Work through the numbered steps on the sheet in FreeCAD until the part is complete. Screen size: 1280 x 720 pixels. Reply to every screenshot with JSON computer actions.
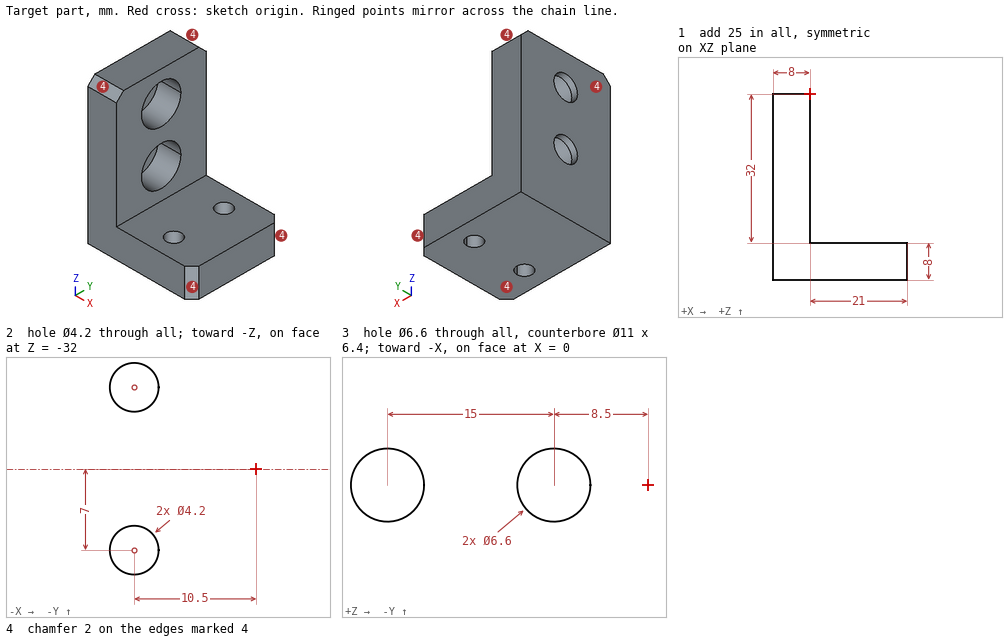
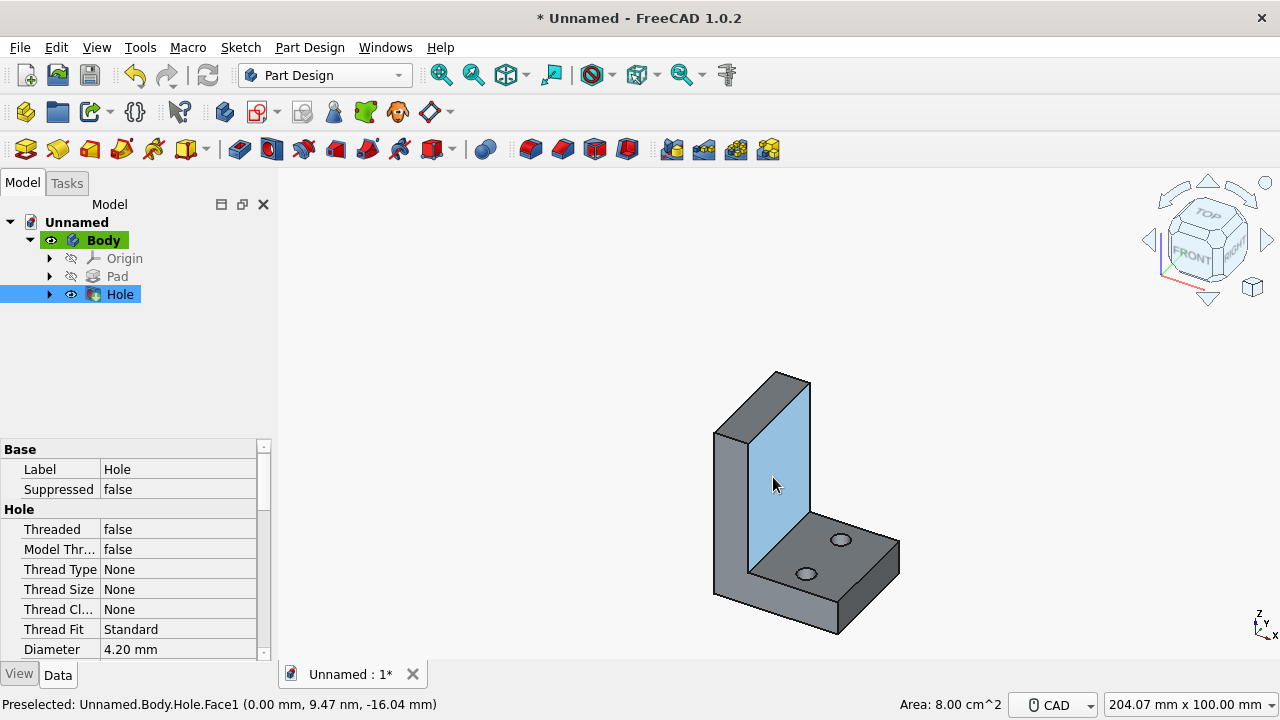
{"action": "left_click", "coordinate": [258, 112]}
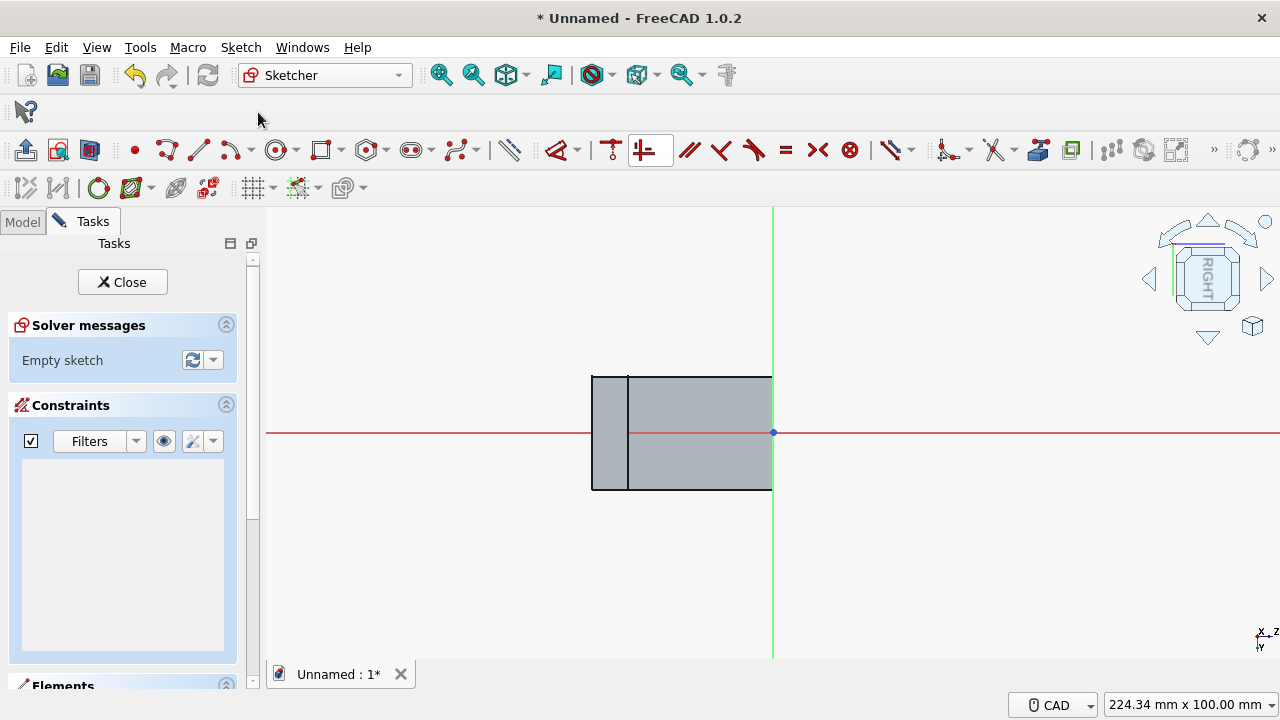
{"action": "left_click", "coordinate": [90, 150]}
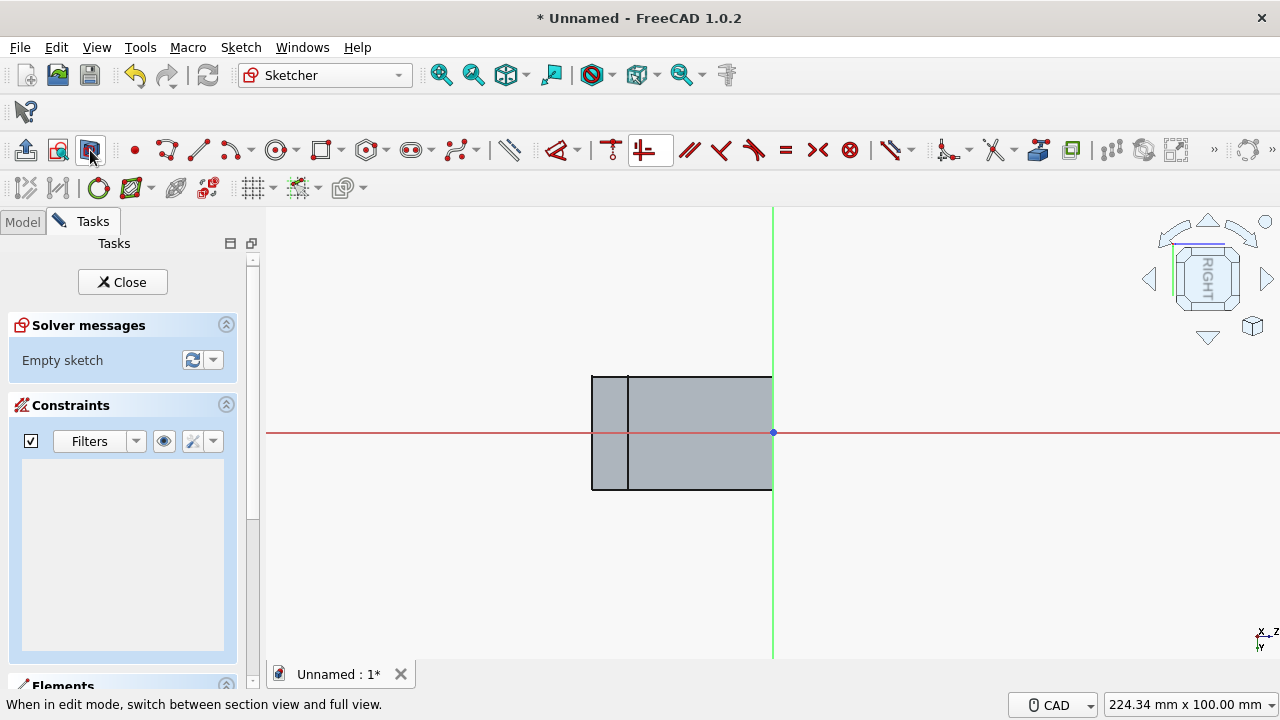
{"action": "scroll", "coordinate": [714, 433], "scroll_direction": "up", "scroll_amount": 8}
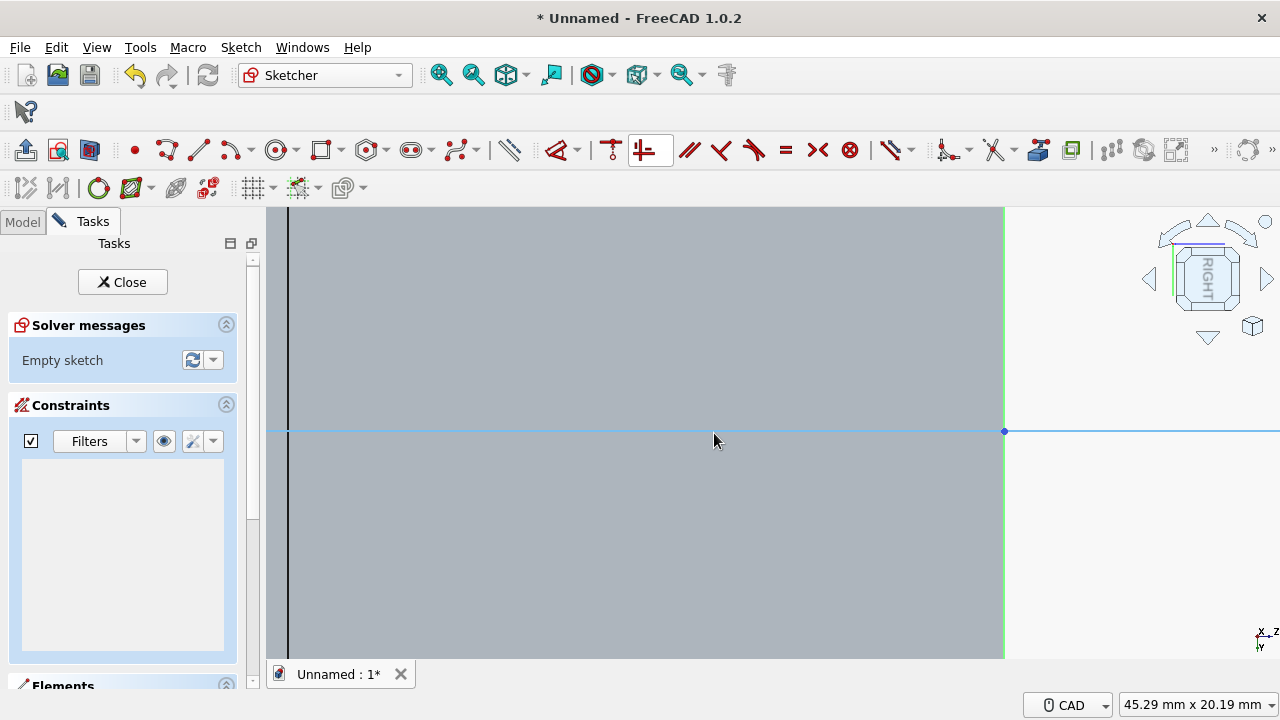
{"action": "key", "text": "g c"}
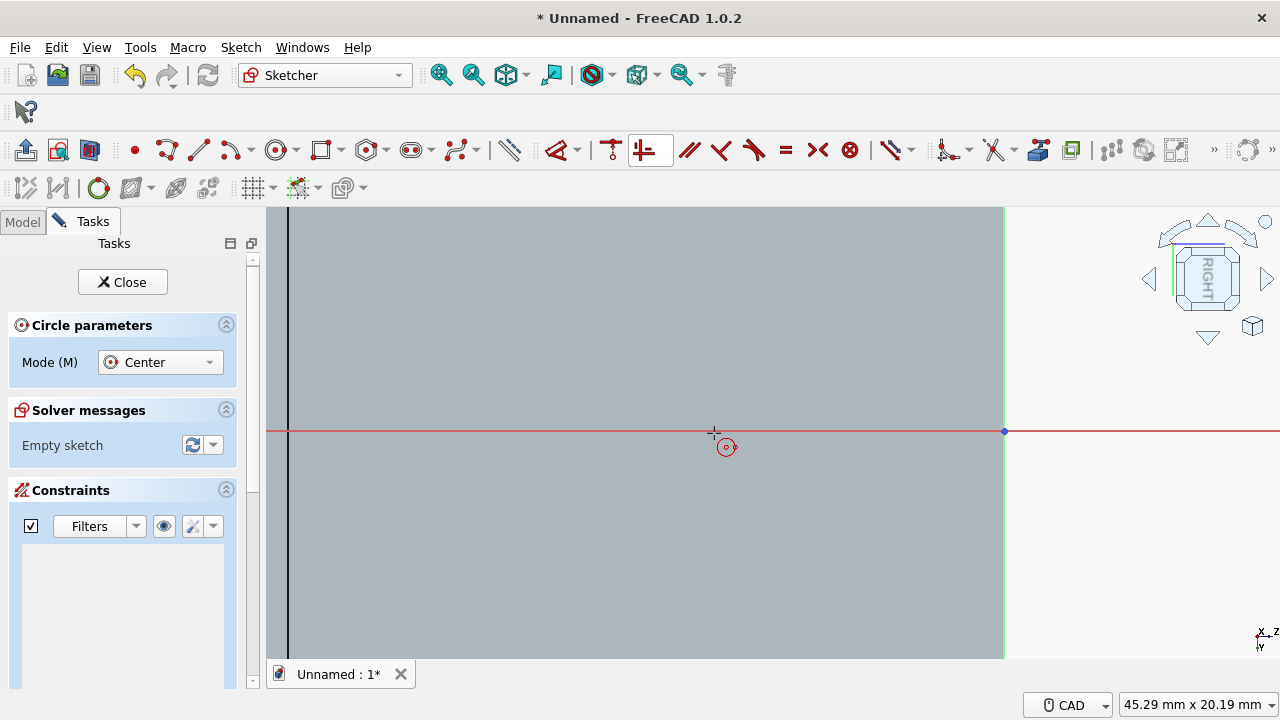
{"action": "left_click", "coordinate": [814, 431]}
{"action": "left_click", "coordinate": [866, 379]}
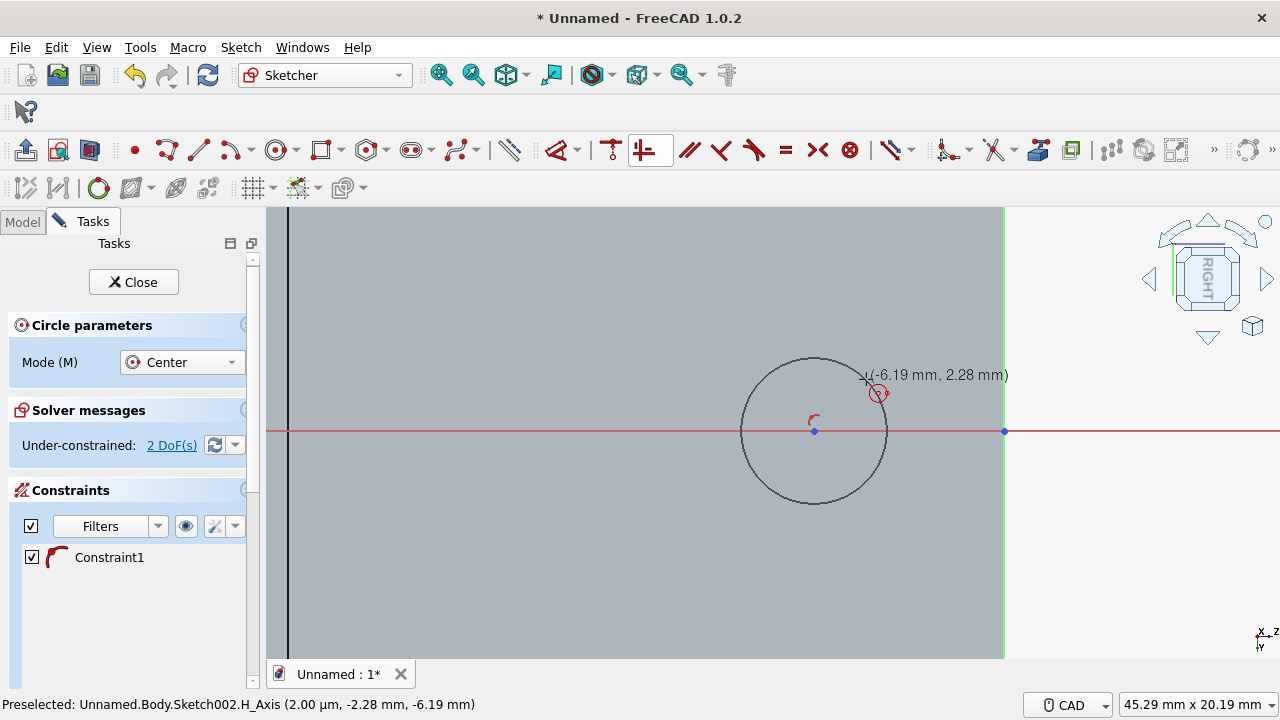
{"action": "left_click", "coordinate": [478, 431]}
{"action": "left_click", "coordinate": [531, 379]}
{"action": "key", "text": "Escape"}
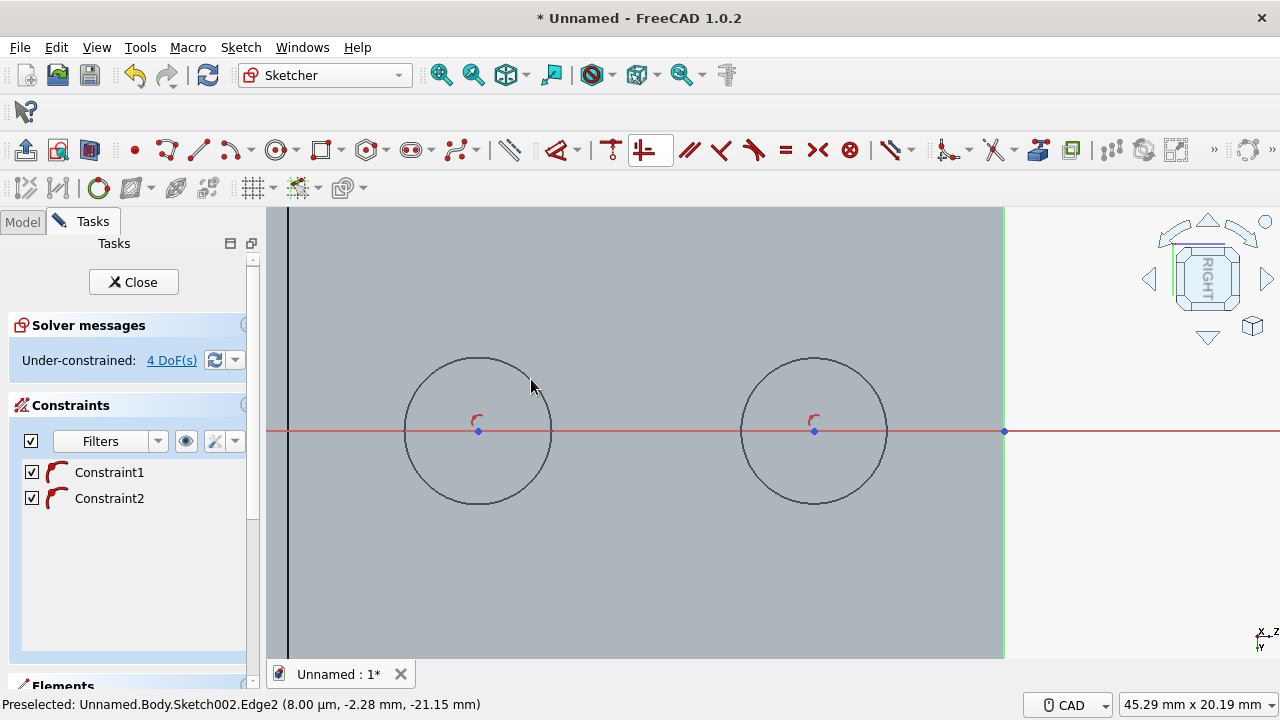
{"action": "left_click", "coordinate": [865, 379]}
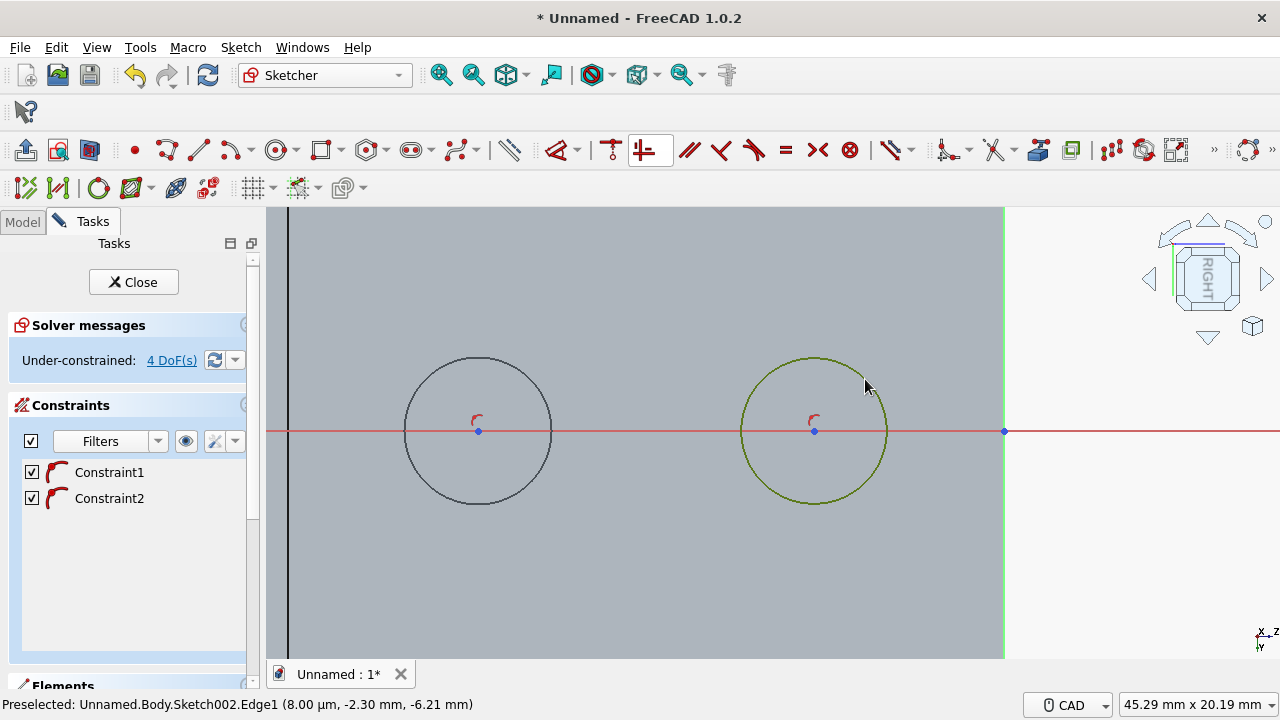
{"action": "left_click", "coordinate": [530, 379]}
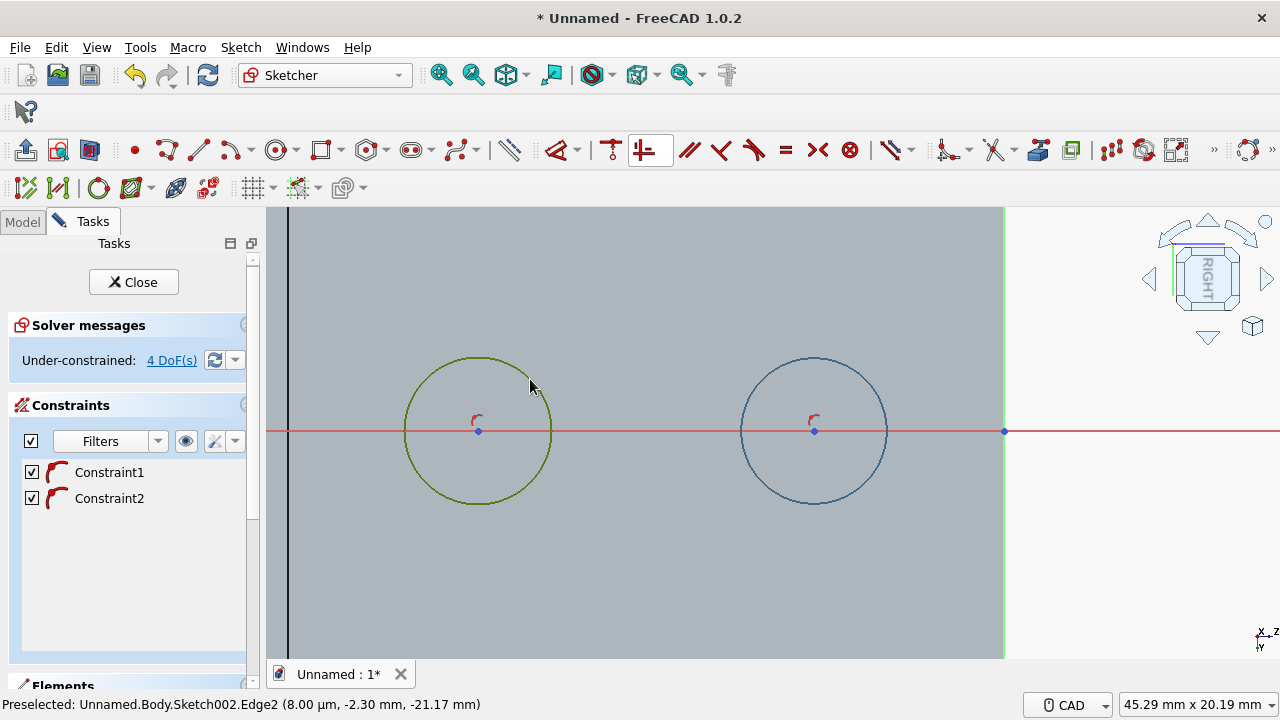
{"action": "left_click", "coordinate": [786, 150]}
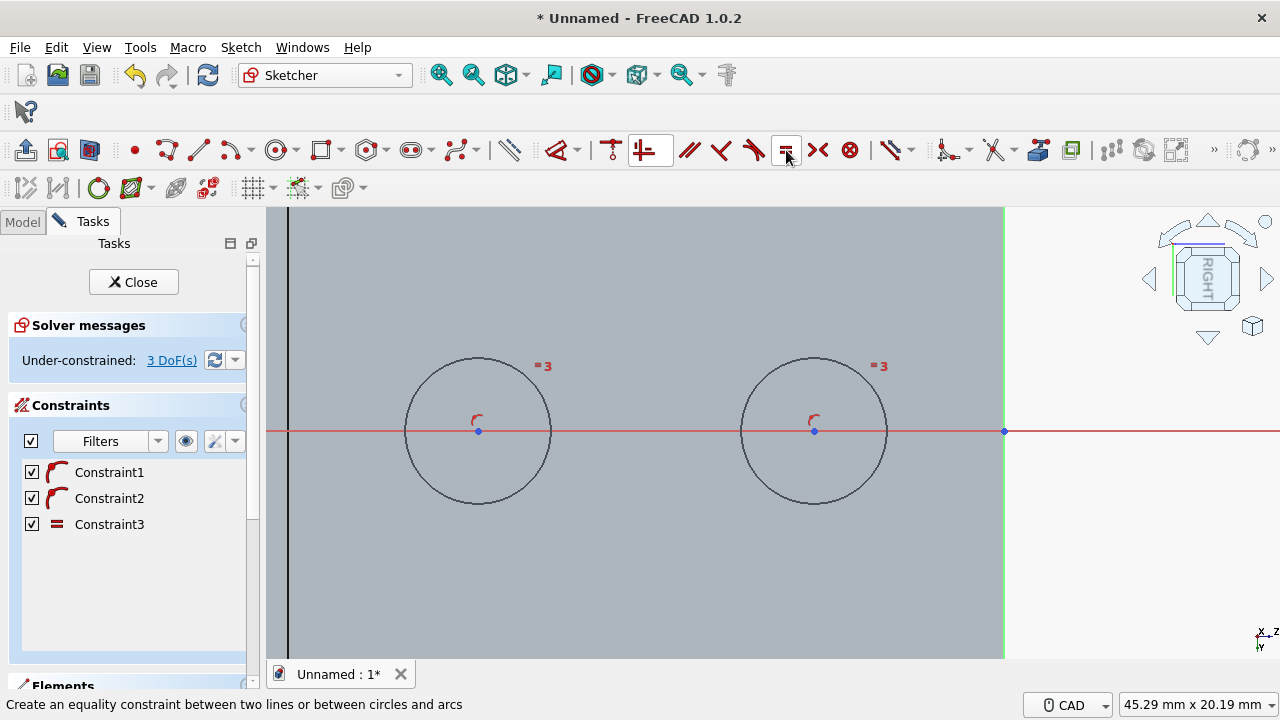
{"action": "left_click", "coordinate": [556, 150]}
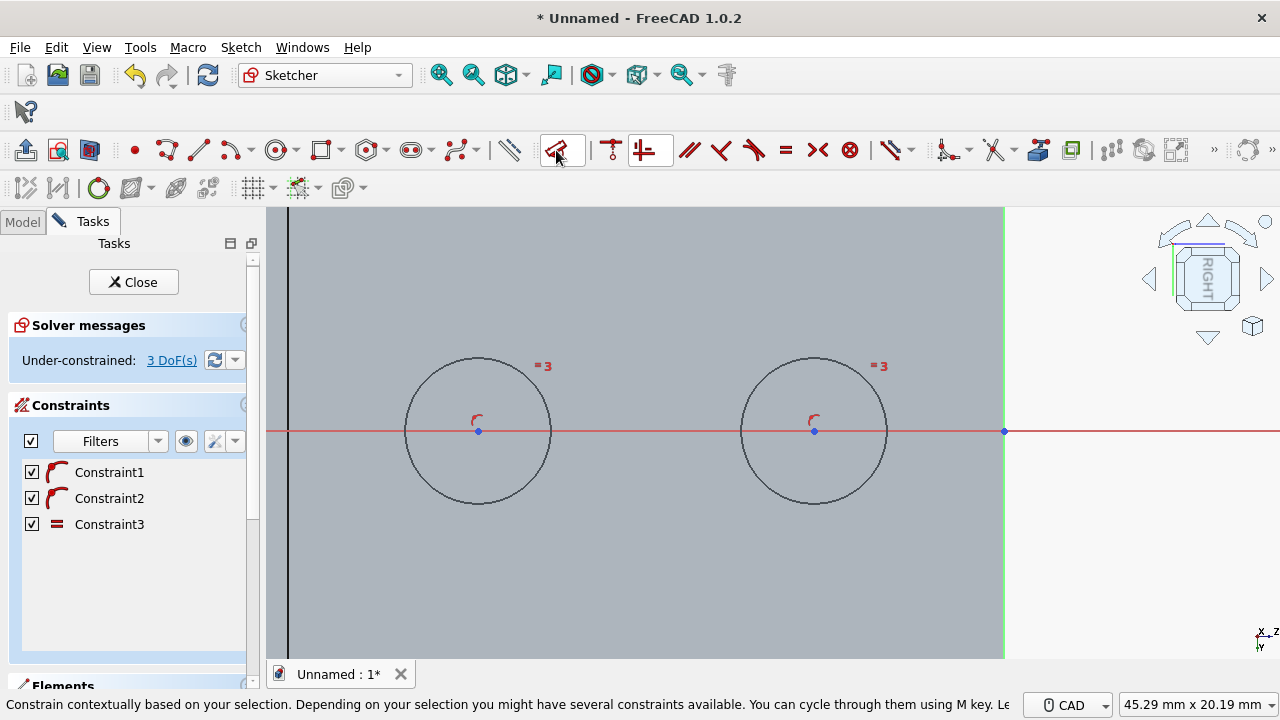
{"action": "left_click", "coordinate": [865, 379]}
{"action": "left_click", "coordinate": [887, 356]}